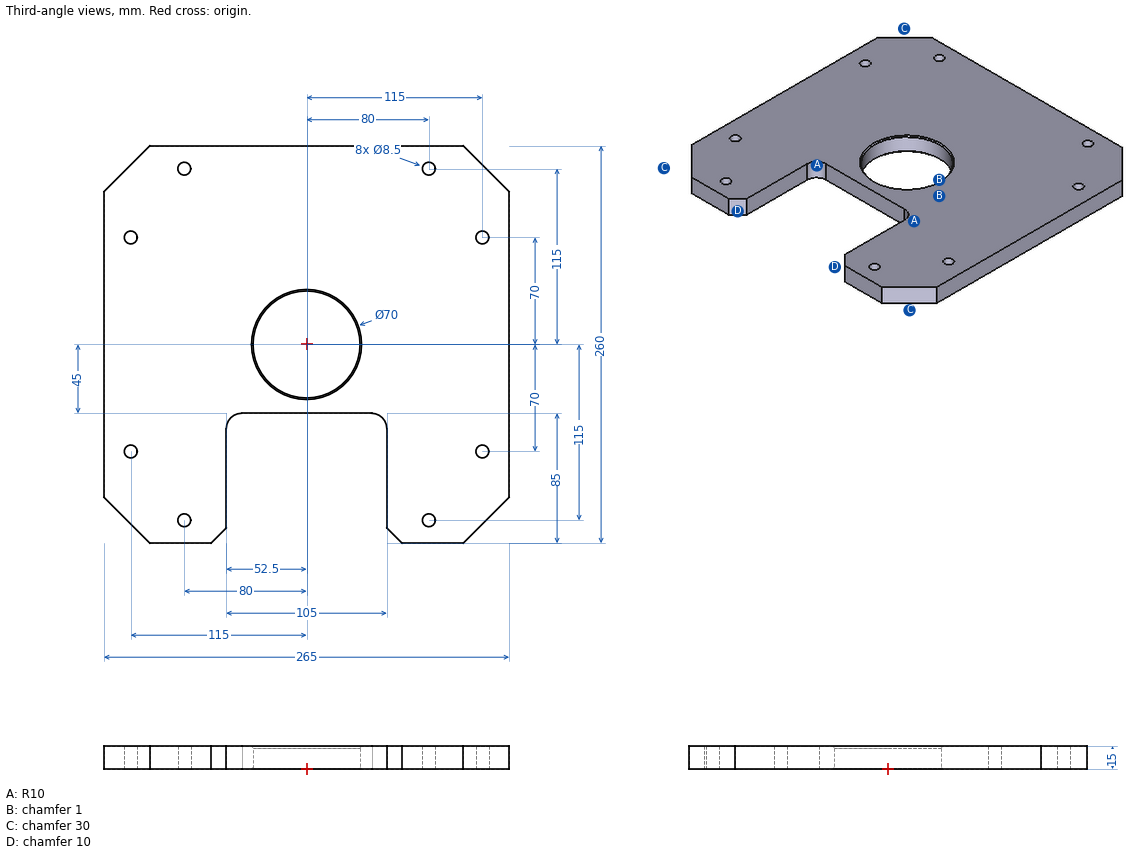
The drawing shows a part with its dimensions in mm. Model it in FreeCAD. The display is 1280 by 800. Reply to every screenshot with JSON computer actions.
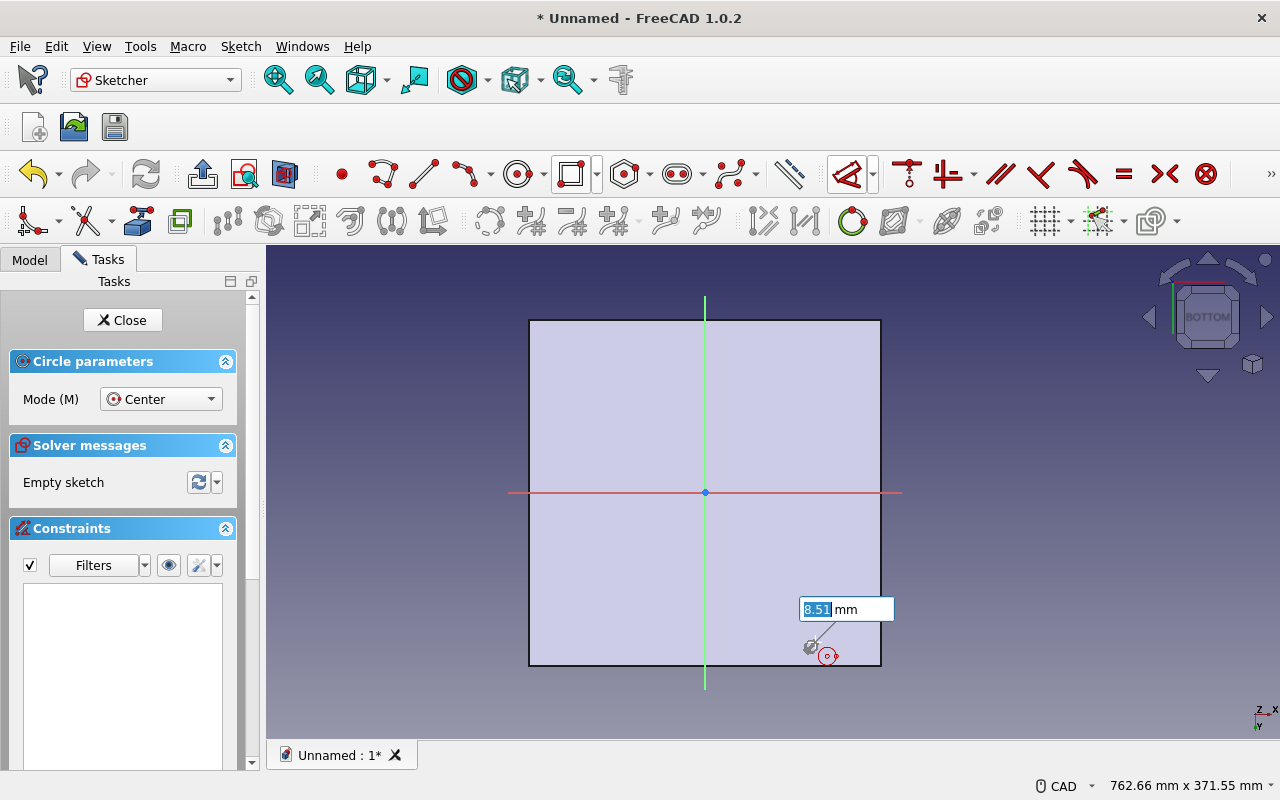
{"action": "type", "text": "8.5"}
{"action": "key", "text": "Return"}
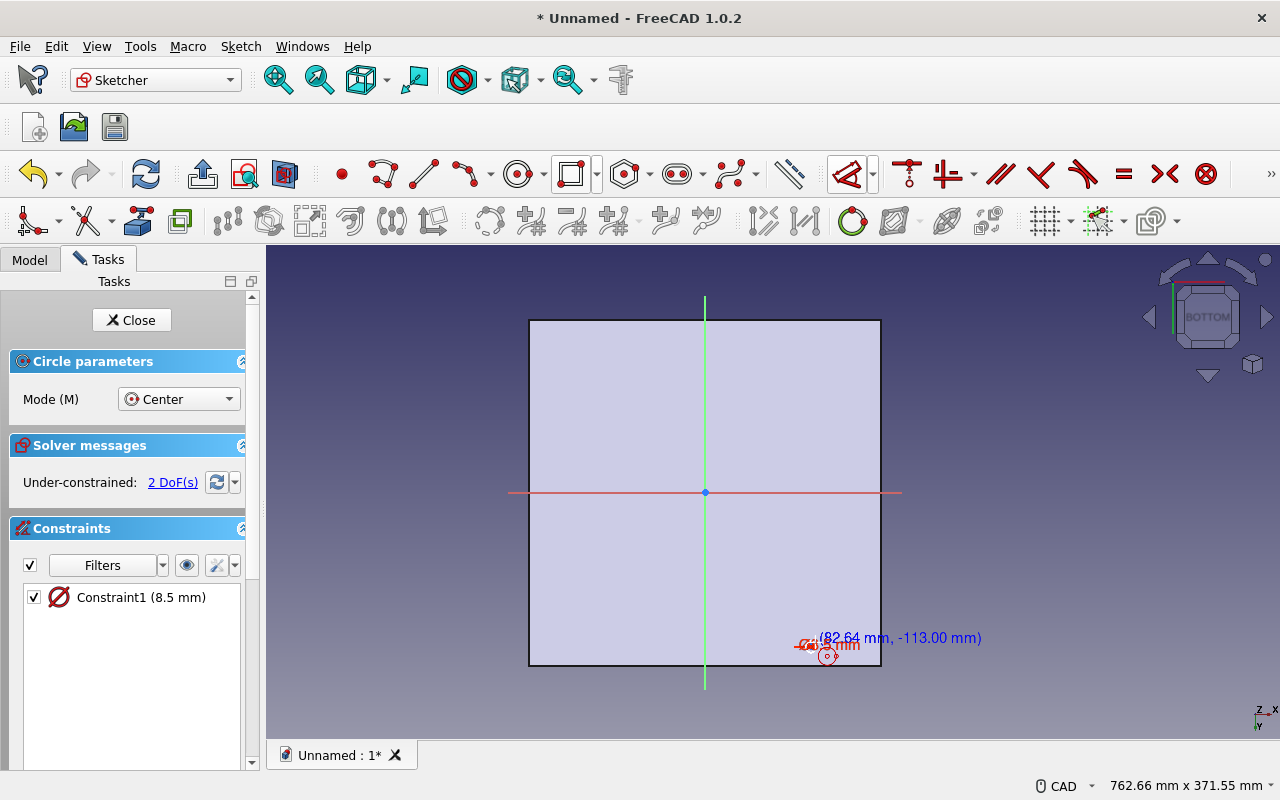
{"action": "scroll", "coordinate": [858, 586], "scroll_direction": "up", "scroll_amount": 7}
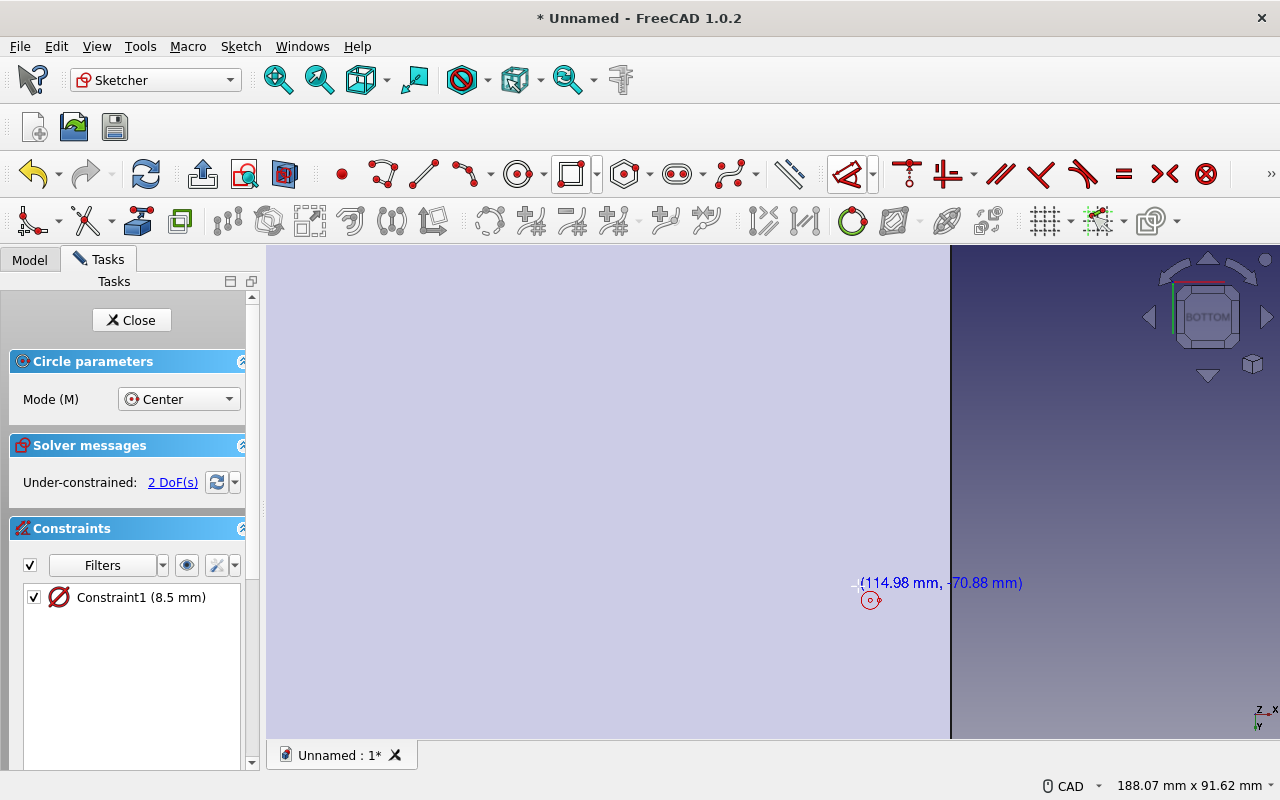
{"action": "scroll", "coordinate": [858, 586], "scroll_direction": "down", "scroll_amount": 7}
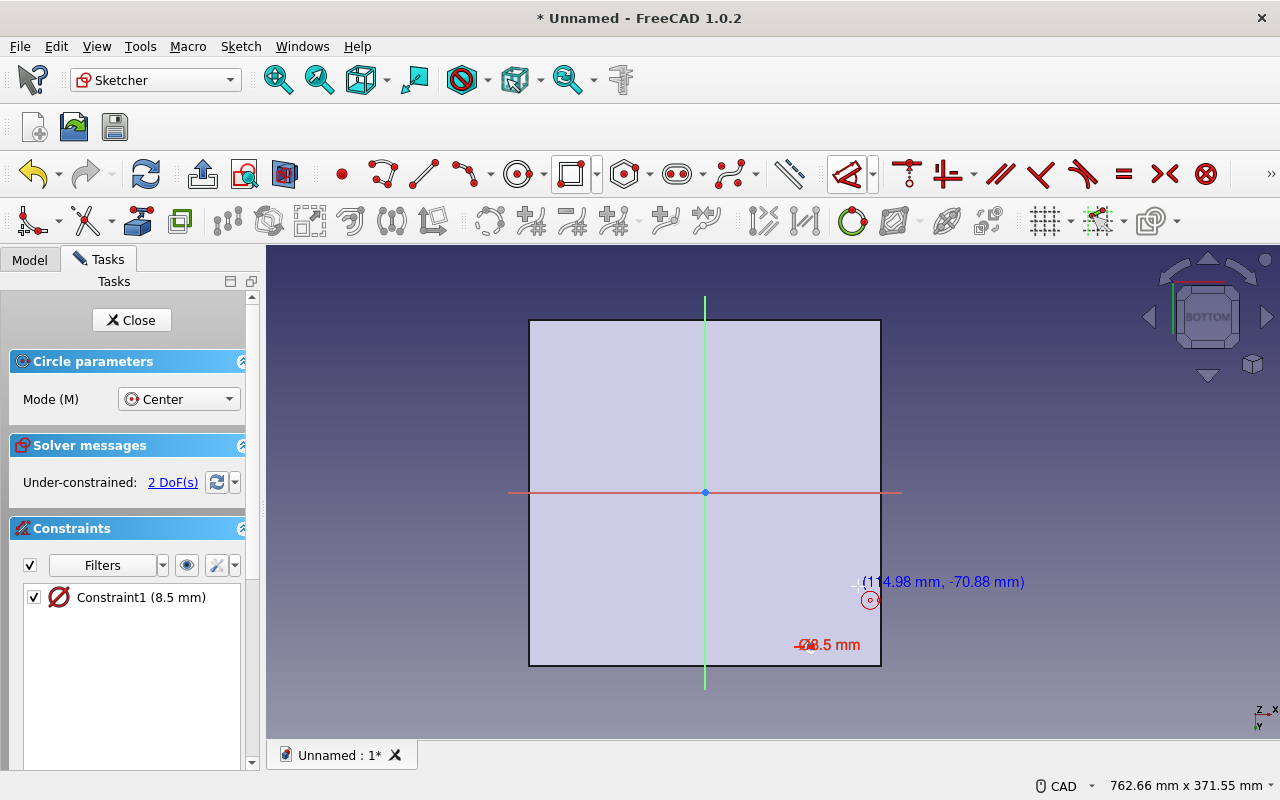
{"action": "left_click", "coordinate": [858, 586]}
{"action": "mouse_move", "coordinate": [862, 582]}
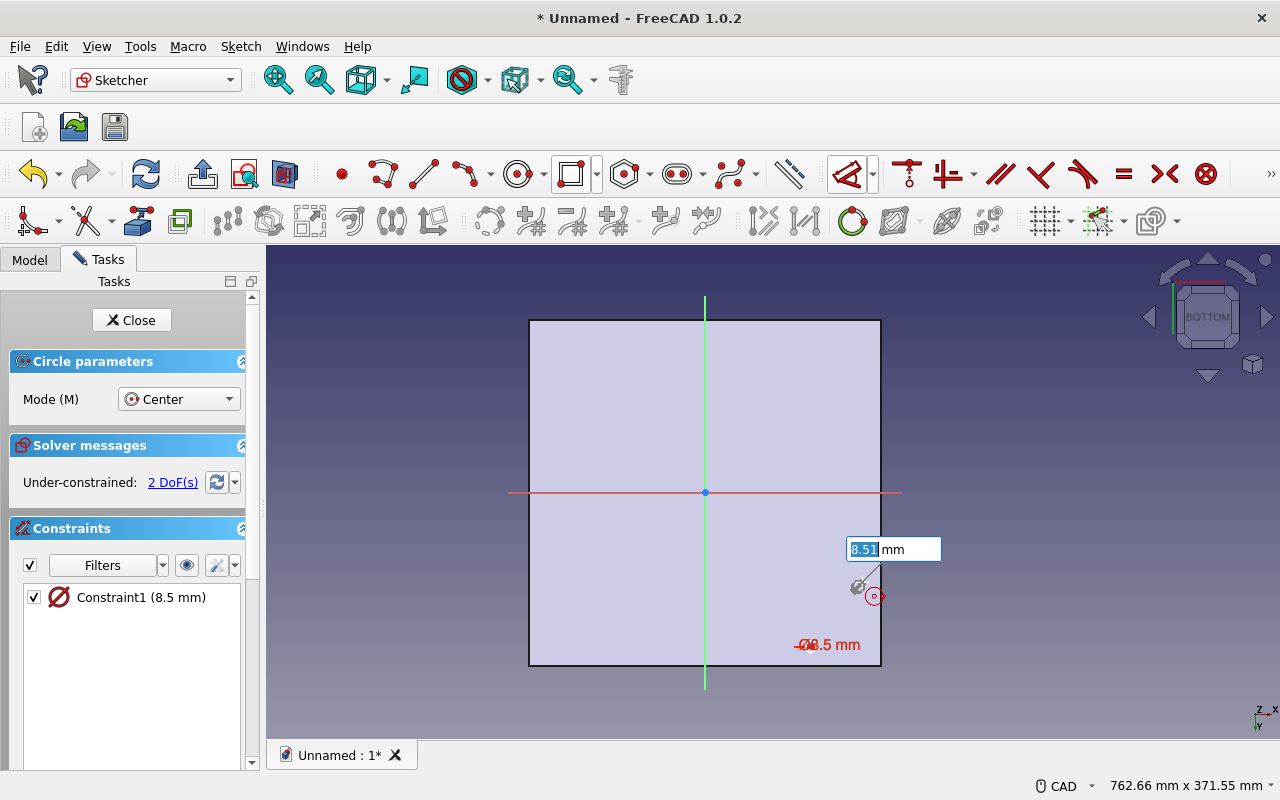
{"action": "type", "text": "8.5"}
{"action": "key", "text": "Return"}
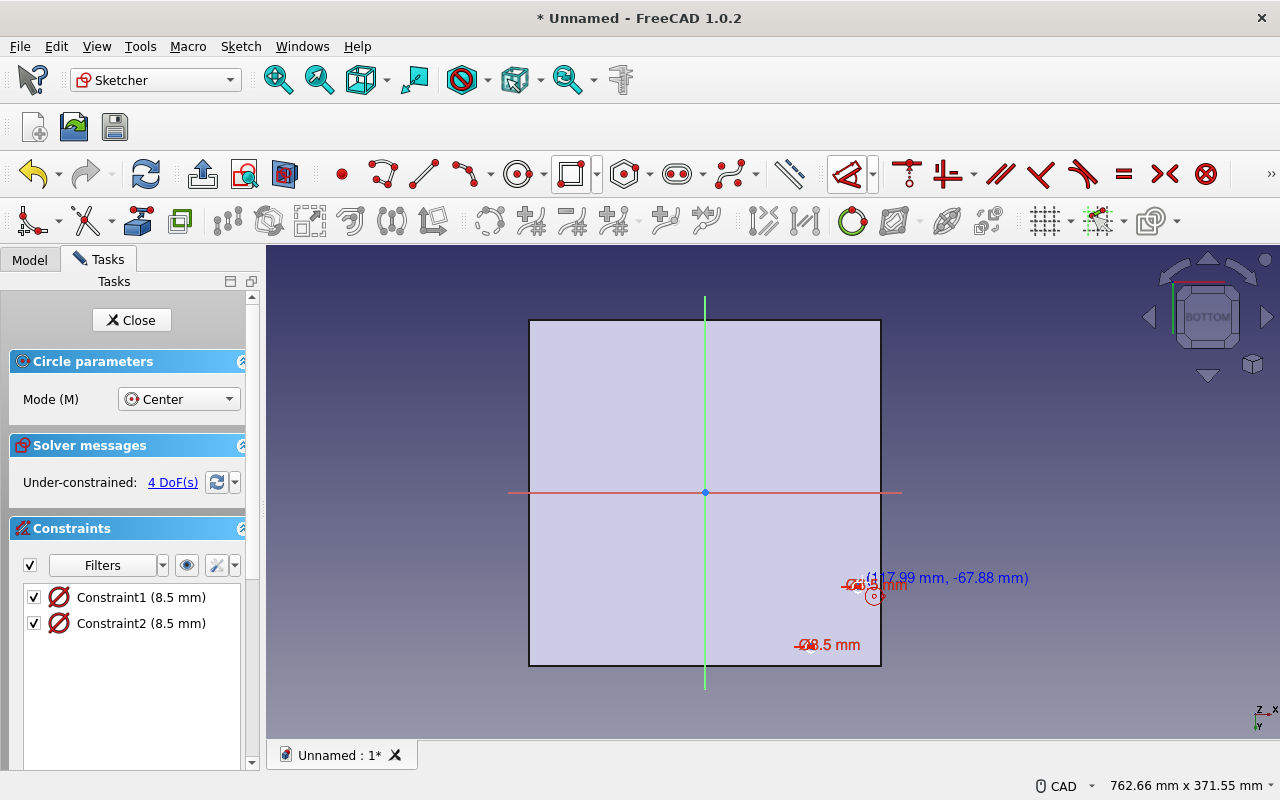
{"action": "scroll", "coordinate": [858, 400], "scroll_direction": "up", "scroll_amount": 7}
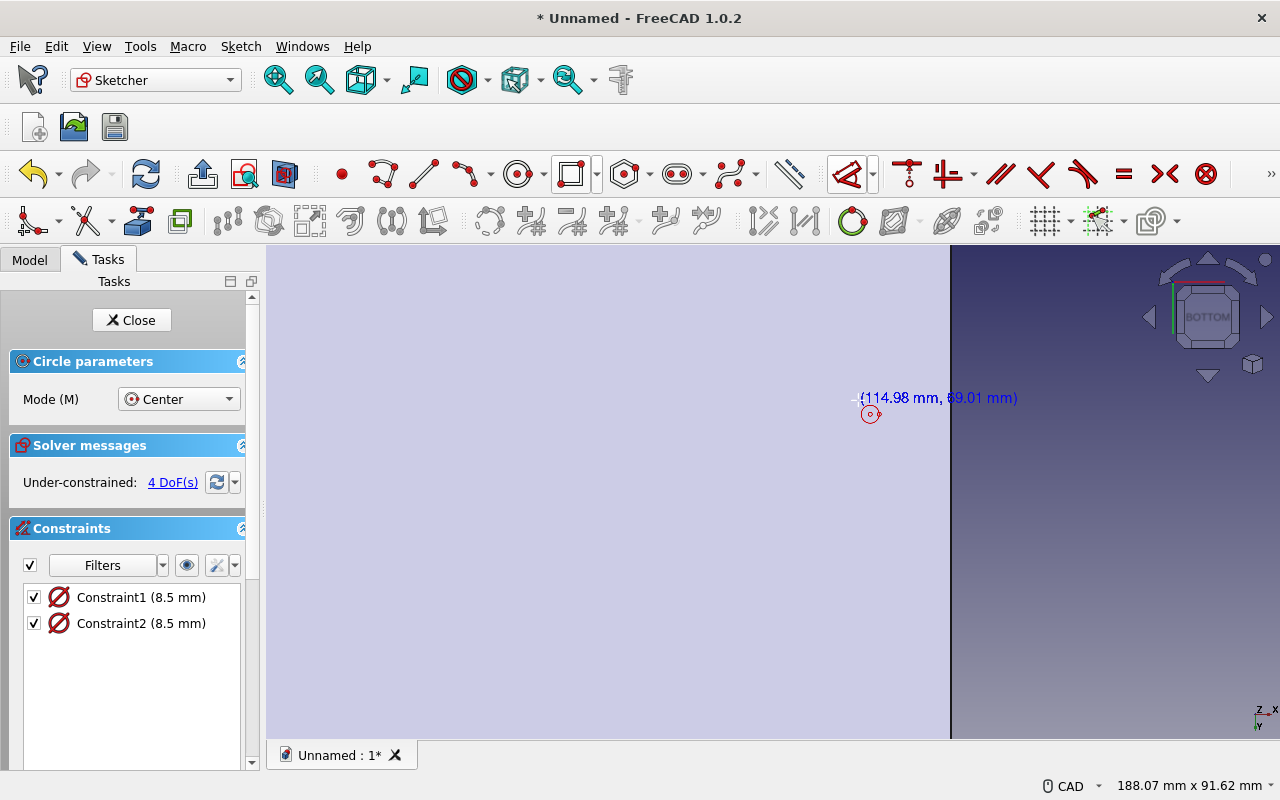
{"action": "scroll", "coordinate": [858, 399], "scroll_direction": "down", "scroll_amount": 7}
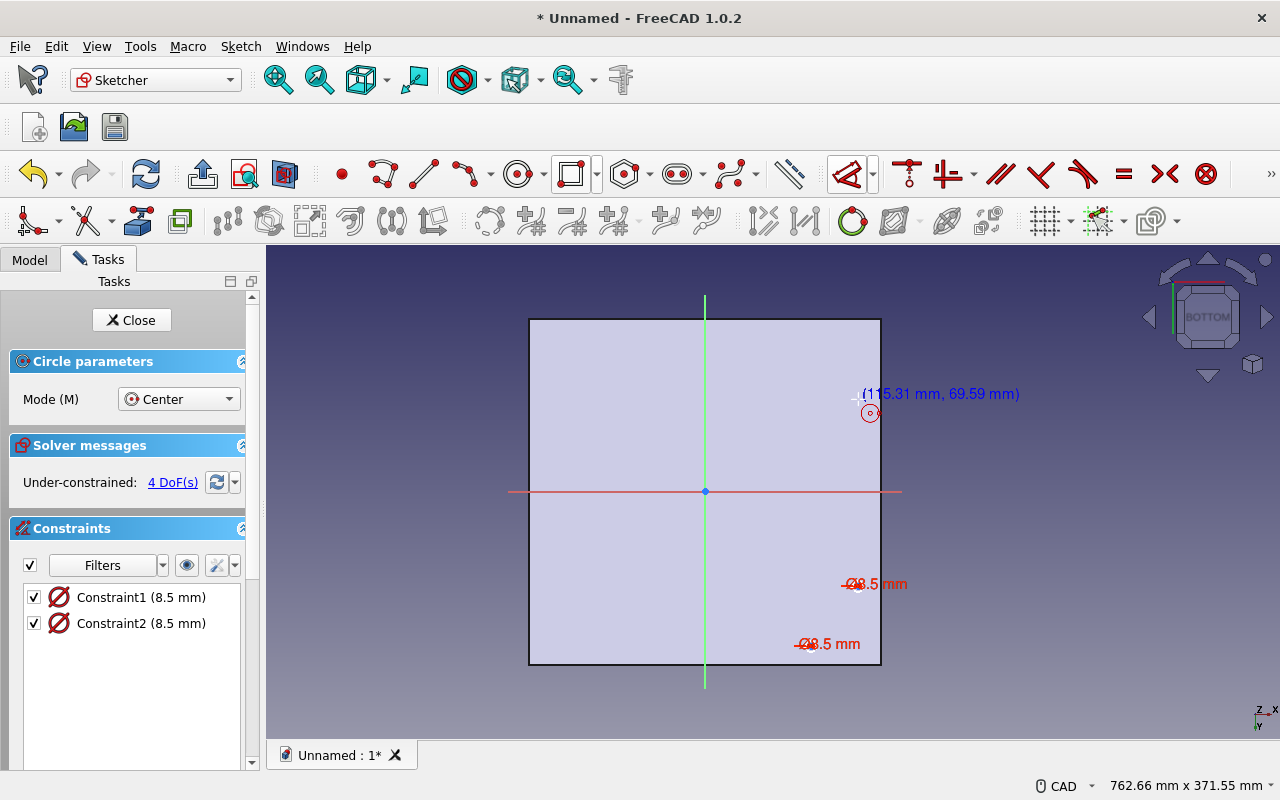
{"action": "left_click", "coordinate": [858, 399]}
{"action": "mouse_move", "coordinate": [862, 395]}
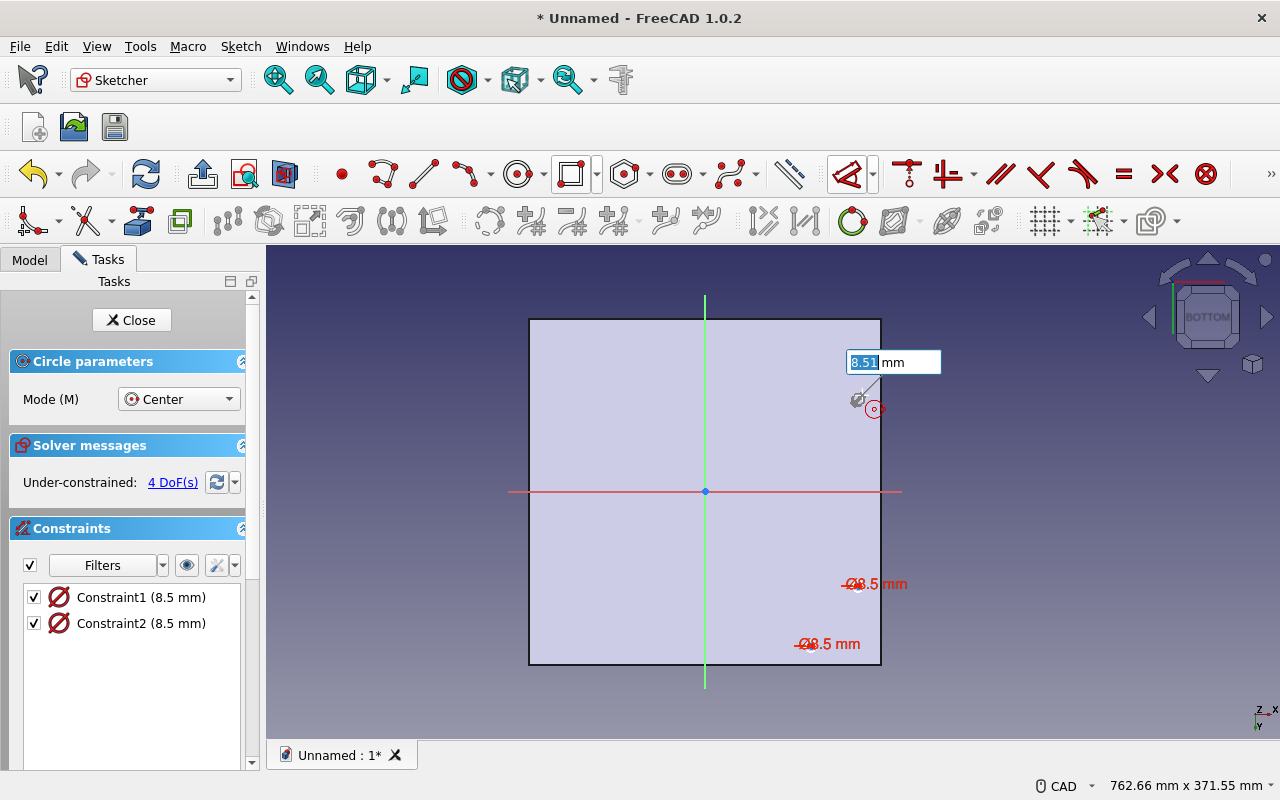
{"action": "type", "text": "8.5"}
{"action": "key", "text": "Return"}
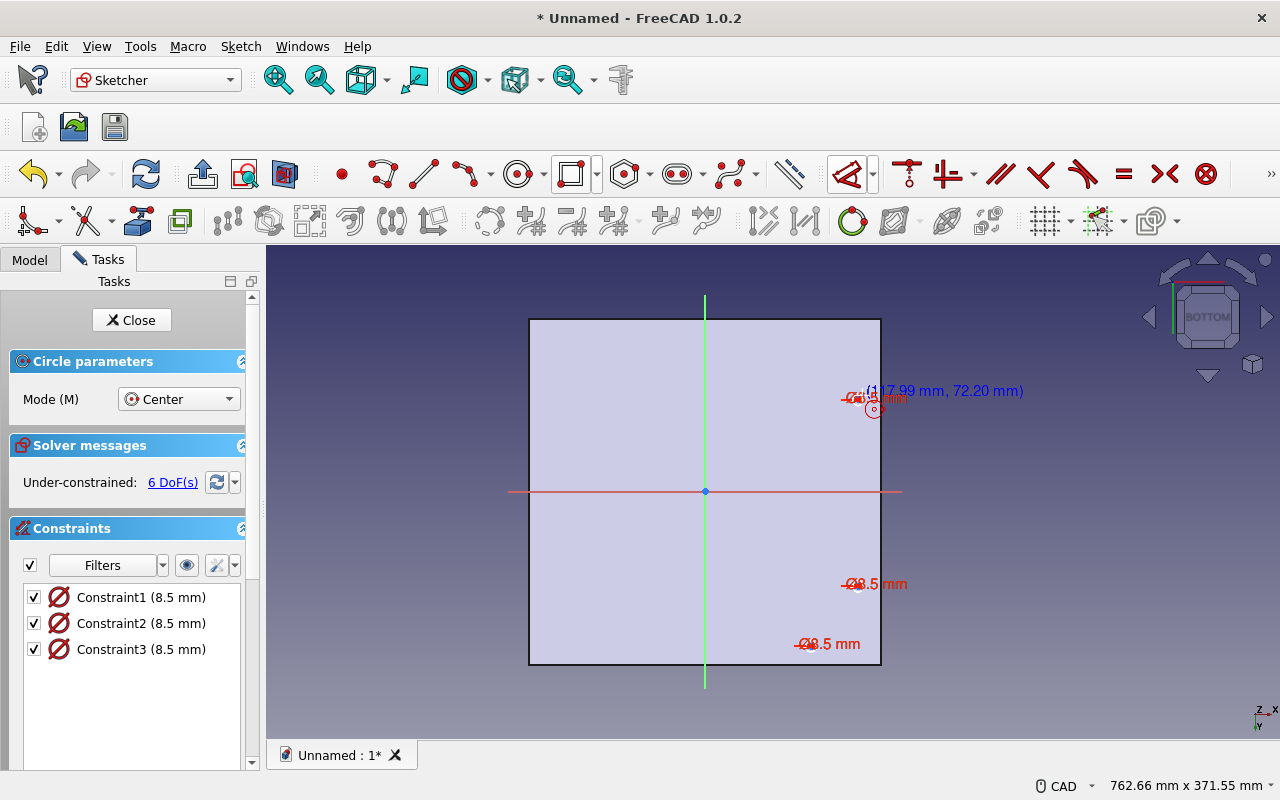
{"action": "scroll", "coordinate": [811, 339], "scroll_direction": "up", "scroll_amount": 7}